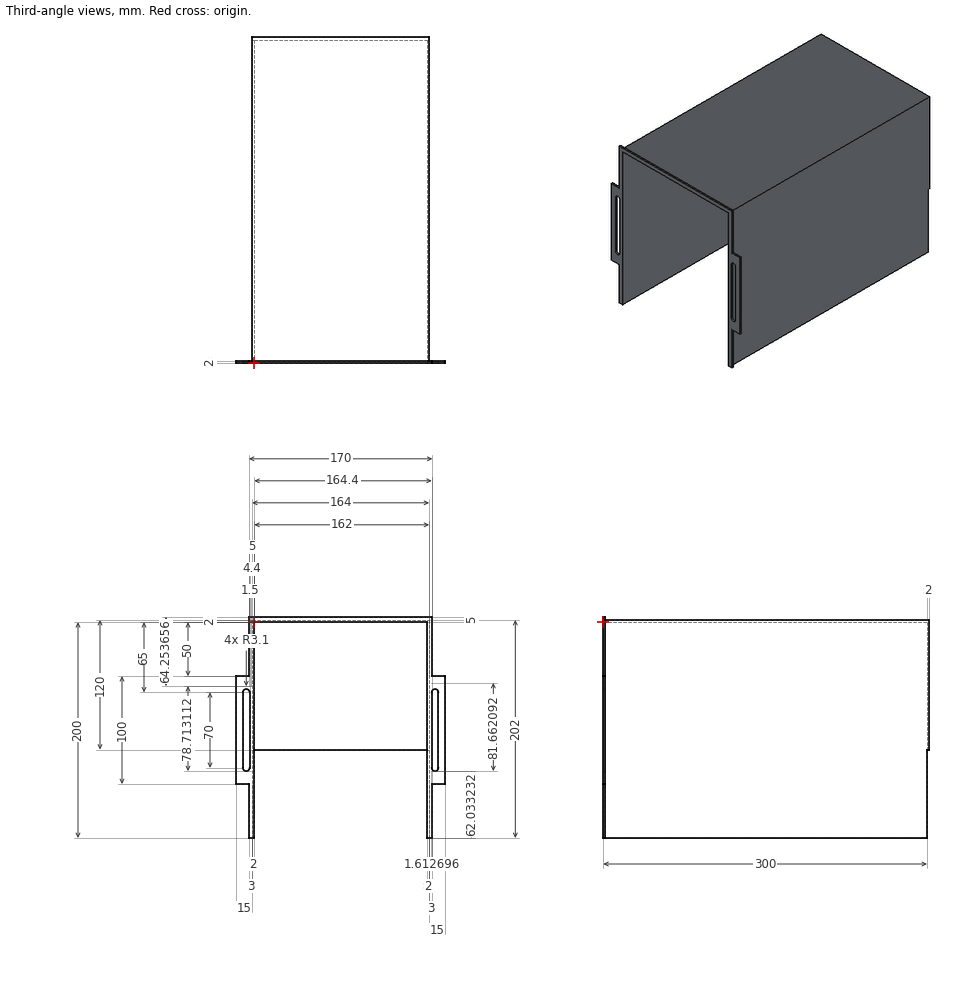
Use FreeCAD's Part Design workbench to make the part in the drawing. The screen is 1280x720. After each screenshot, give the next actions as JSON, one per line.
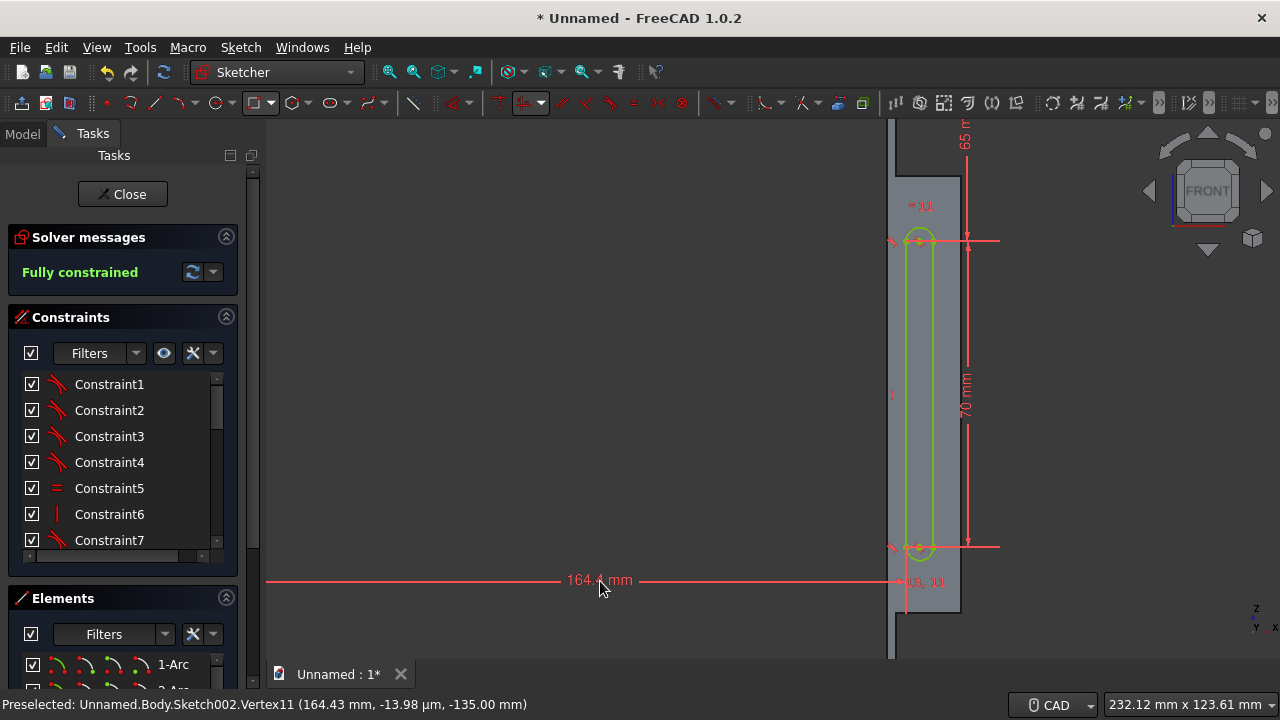
{"action": "left_click", "coordinate": [123, 194]}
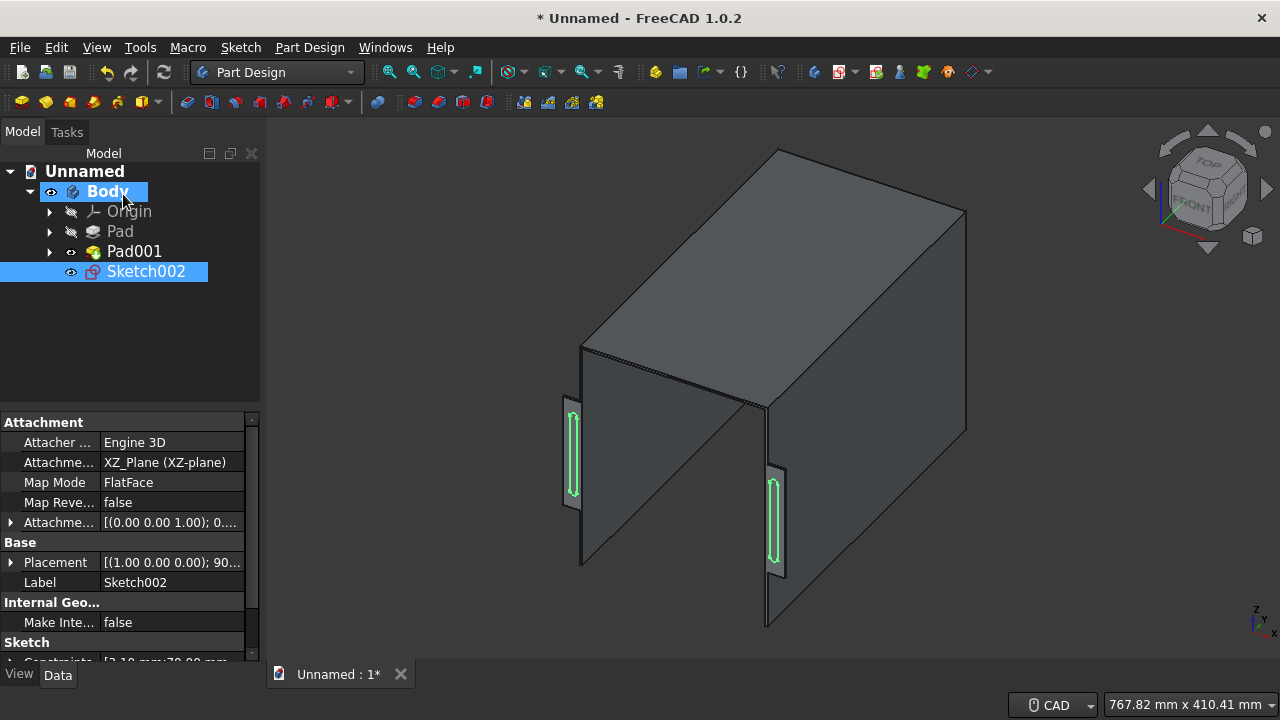
{"action": "left_click", "coordinate": [188, 102]}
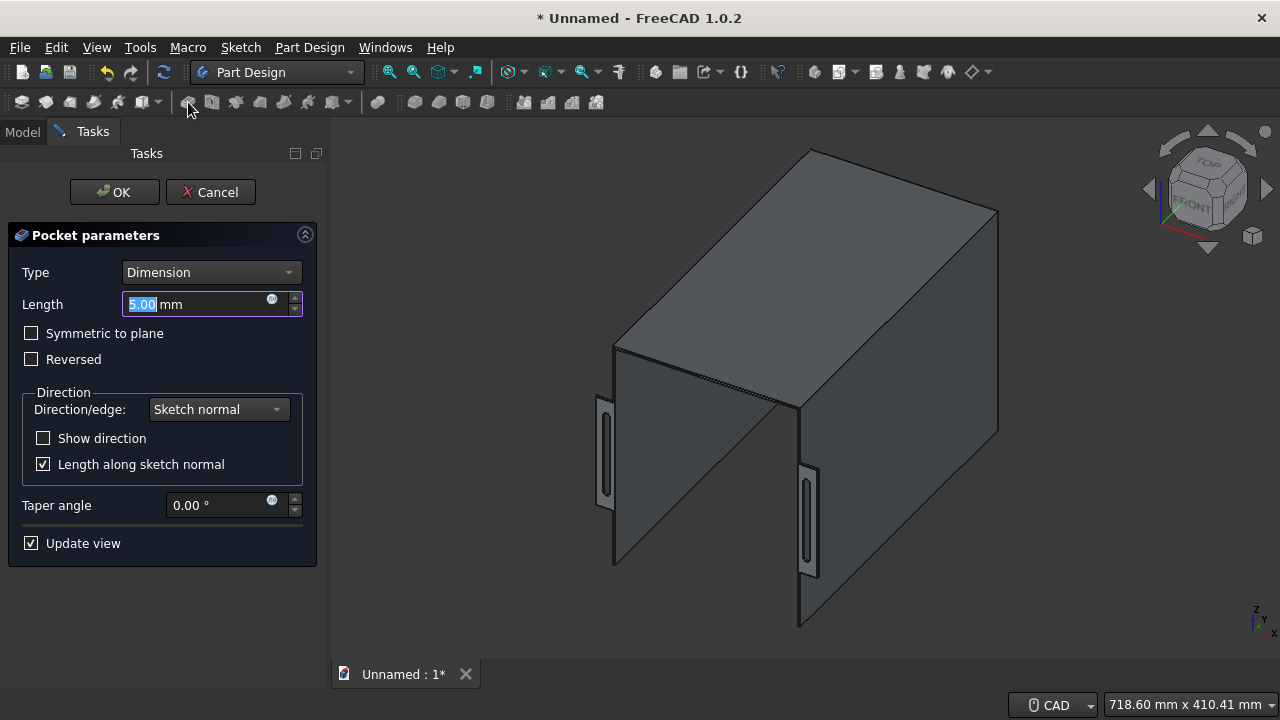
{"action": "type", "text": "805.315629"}
{"action": "key", "text": "Tab"}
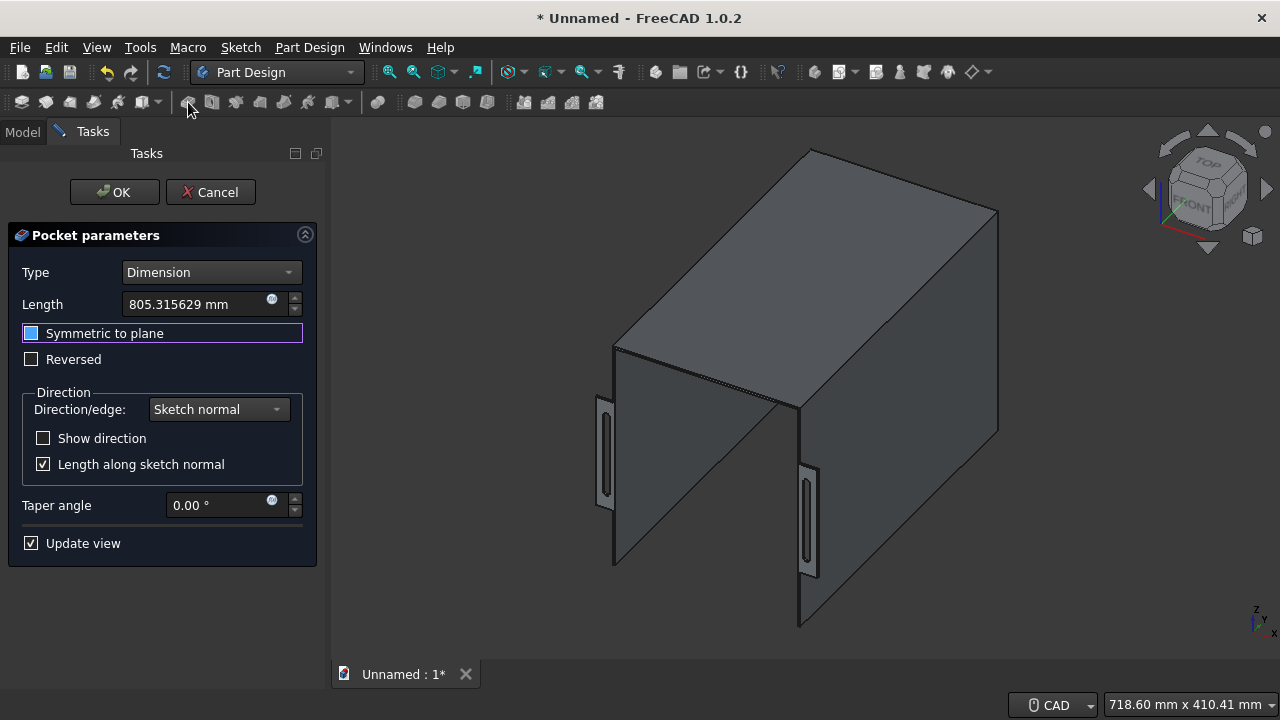
{"action": "left_click", "coordinate": [30, 333]}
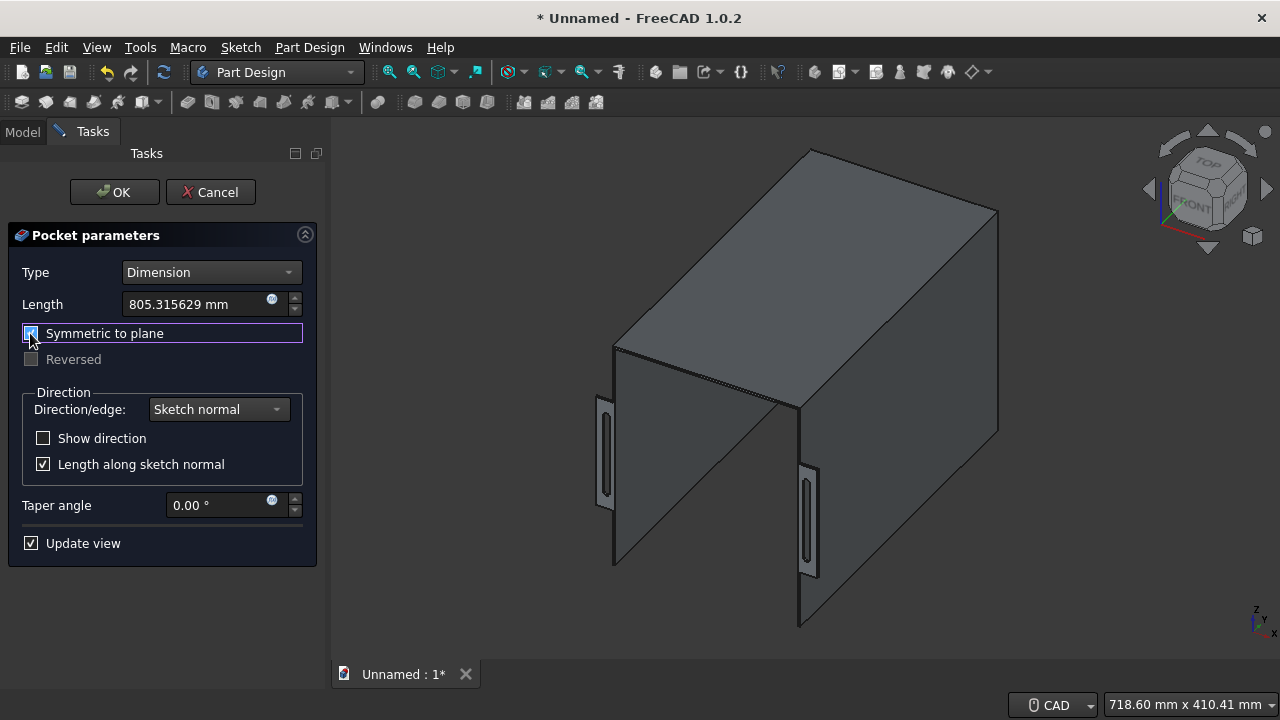
{"action": "left_click", "coordinate": [115, 192]}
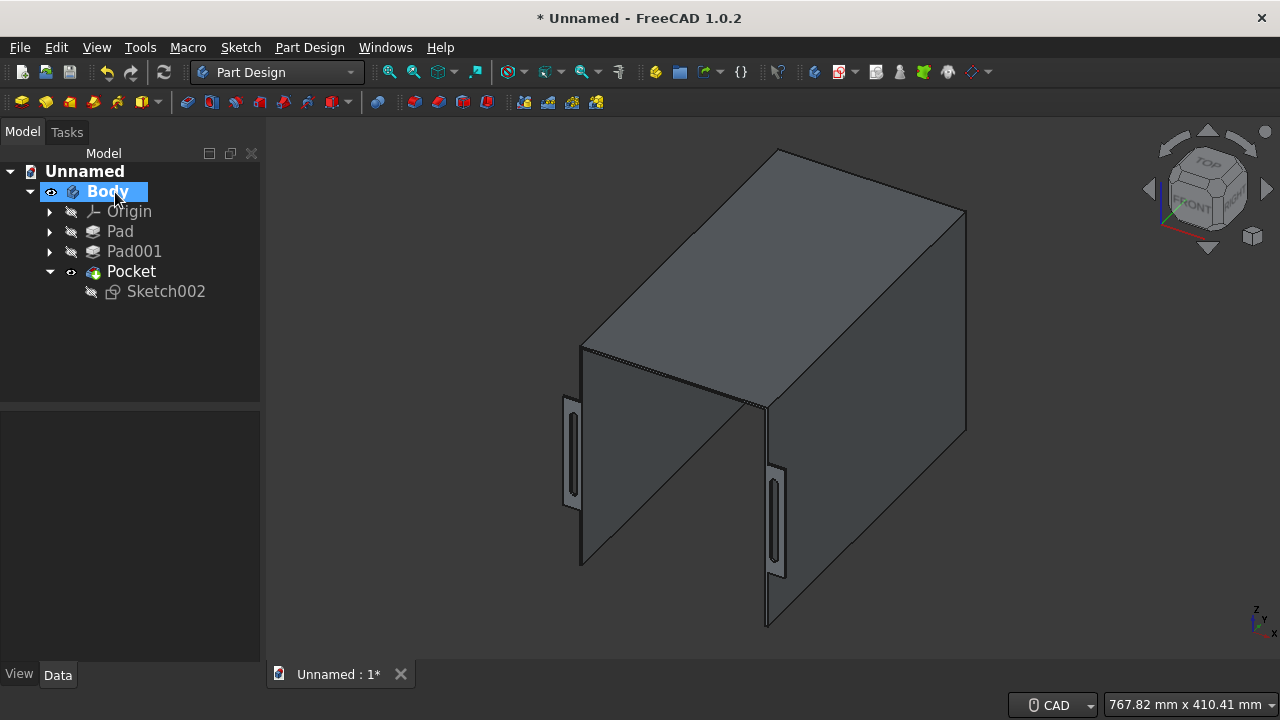
{"action": "key", "text": "4"}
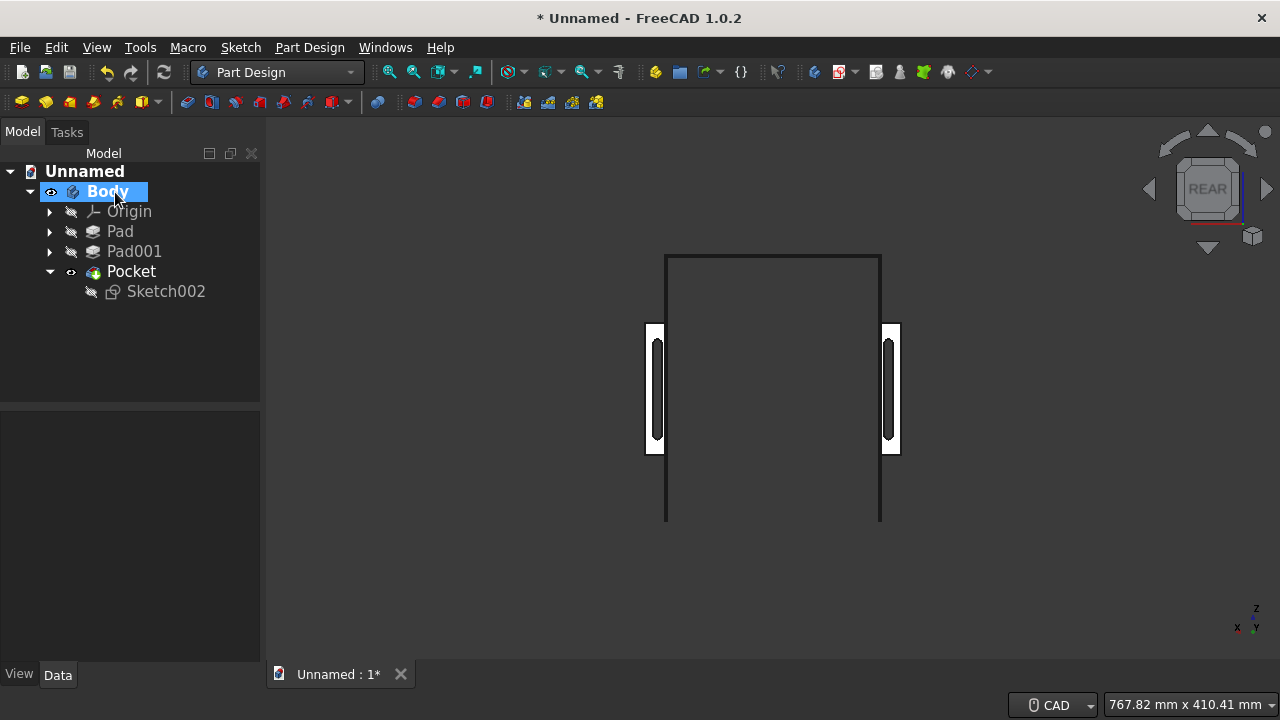
{"action": "scroll", "coordinate": [808, 254], "scroll_direction": "up", "scroll_amount": 14}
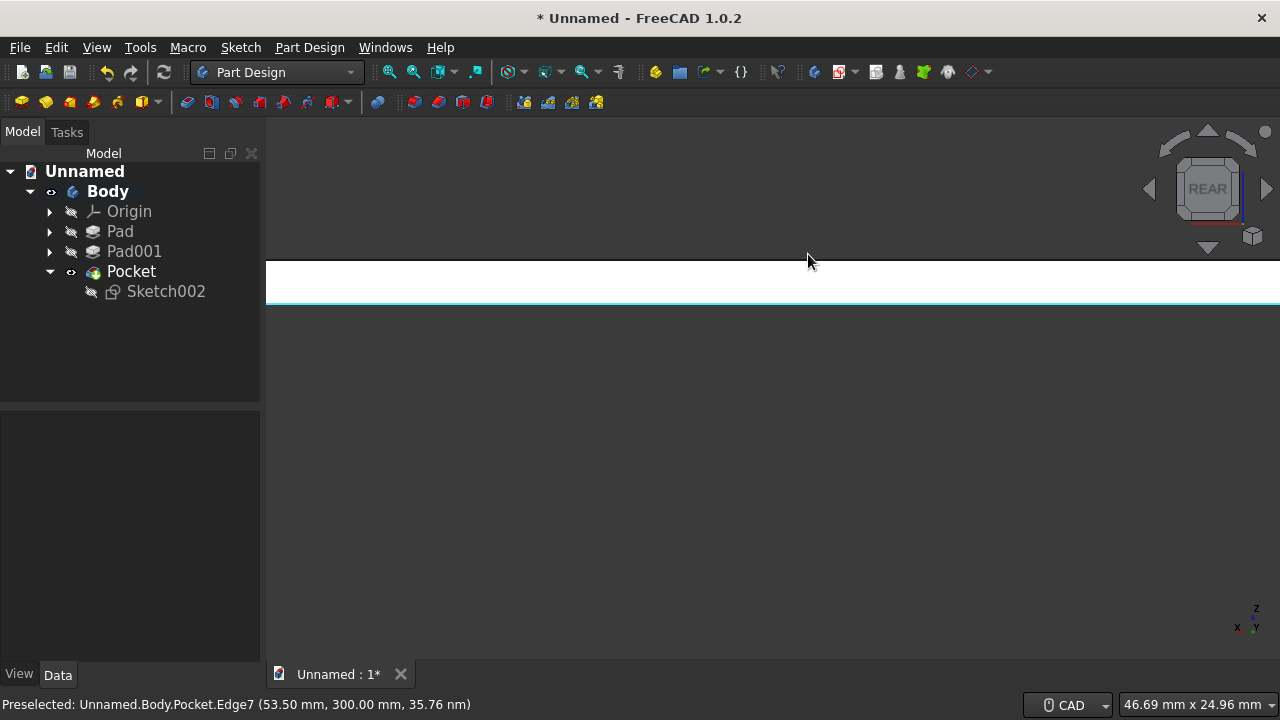
{"action": "left_click", "coordinate": [803, 274]}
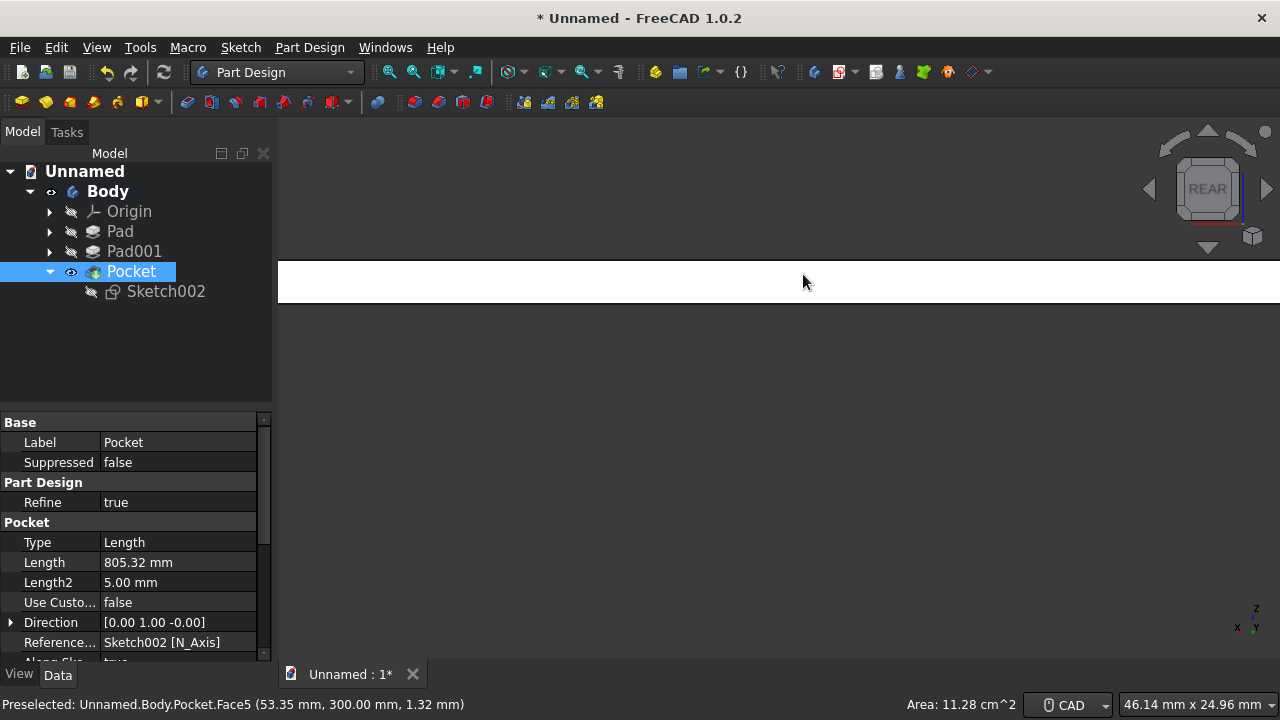
{"action": "left_click", "coordinate": [840, 72]}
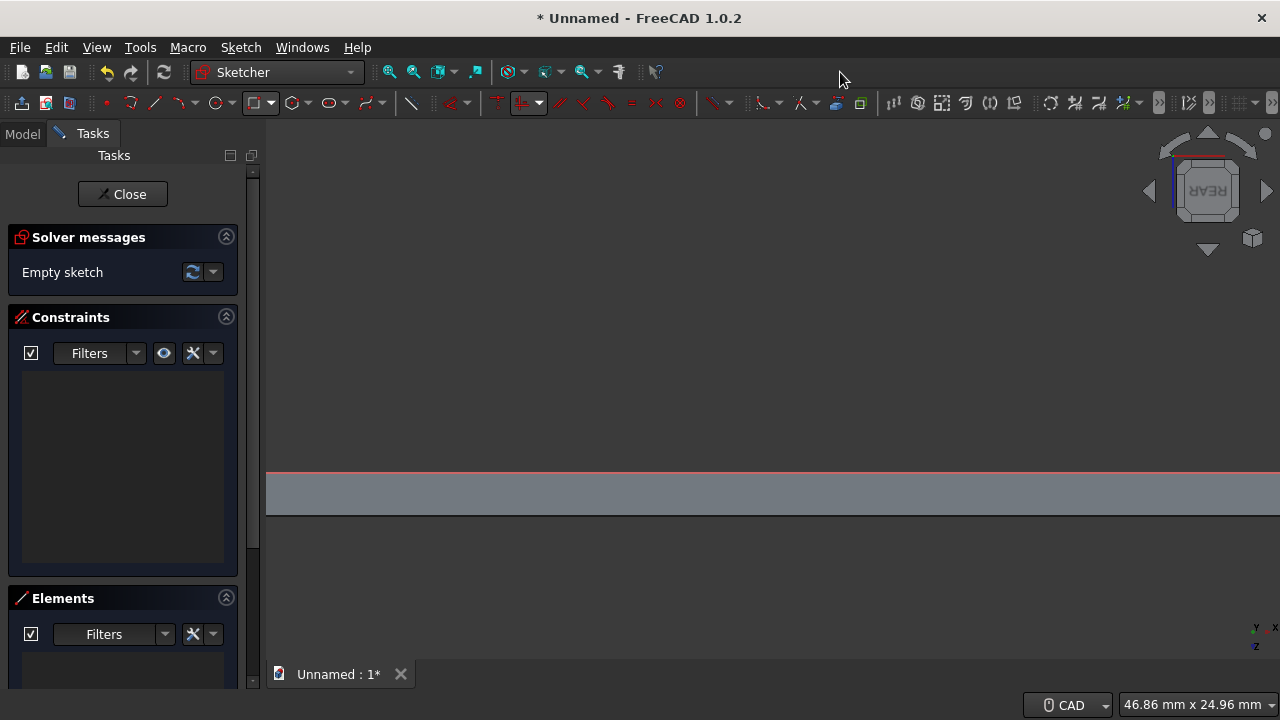
{"action": "scroll", "coordinate": [608, 572], "scroll_direction": "down", "scroll_amount": 10}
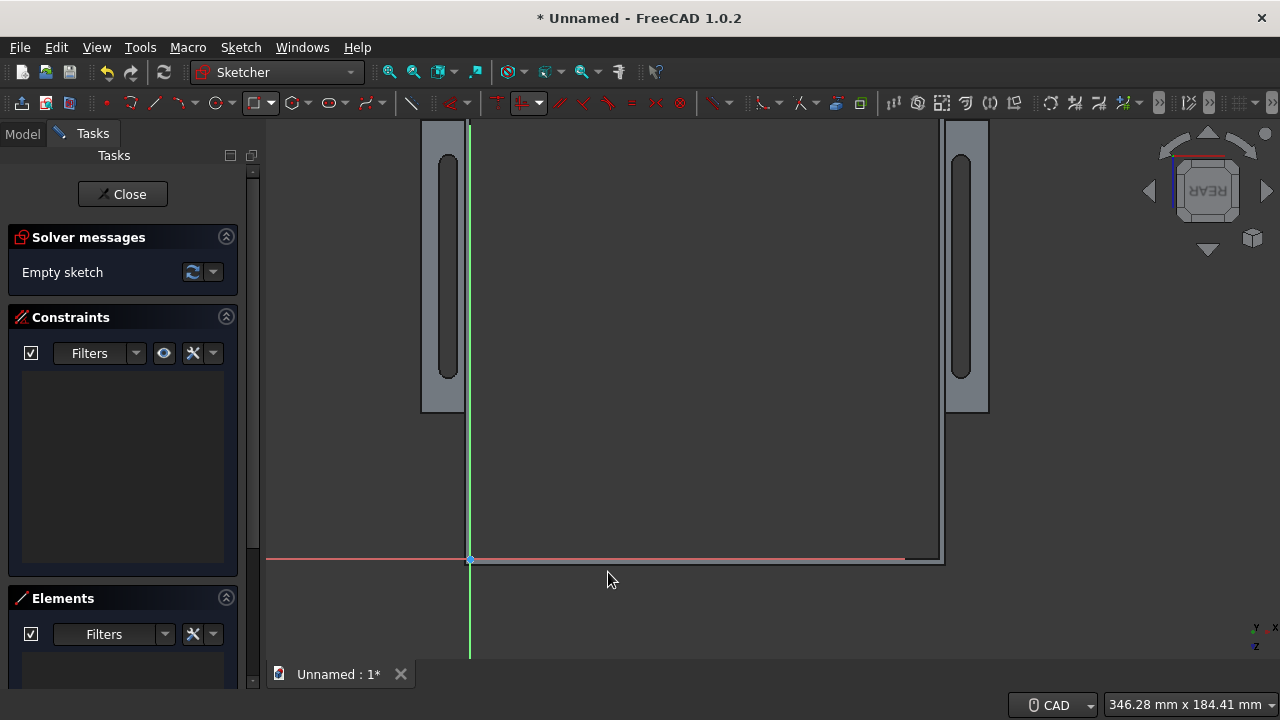
{"action": "left_click", "coordinate": [254, 104]}